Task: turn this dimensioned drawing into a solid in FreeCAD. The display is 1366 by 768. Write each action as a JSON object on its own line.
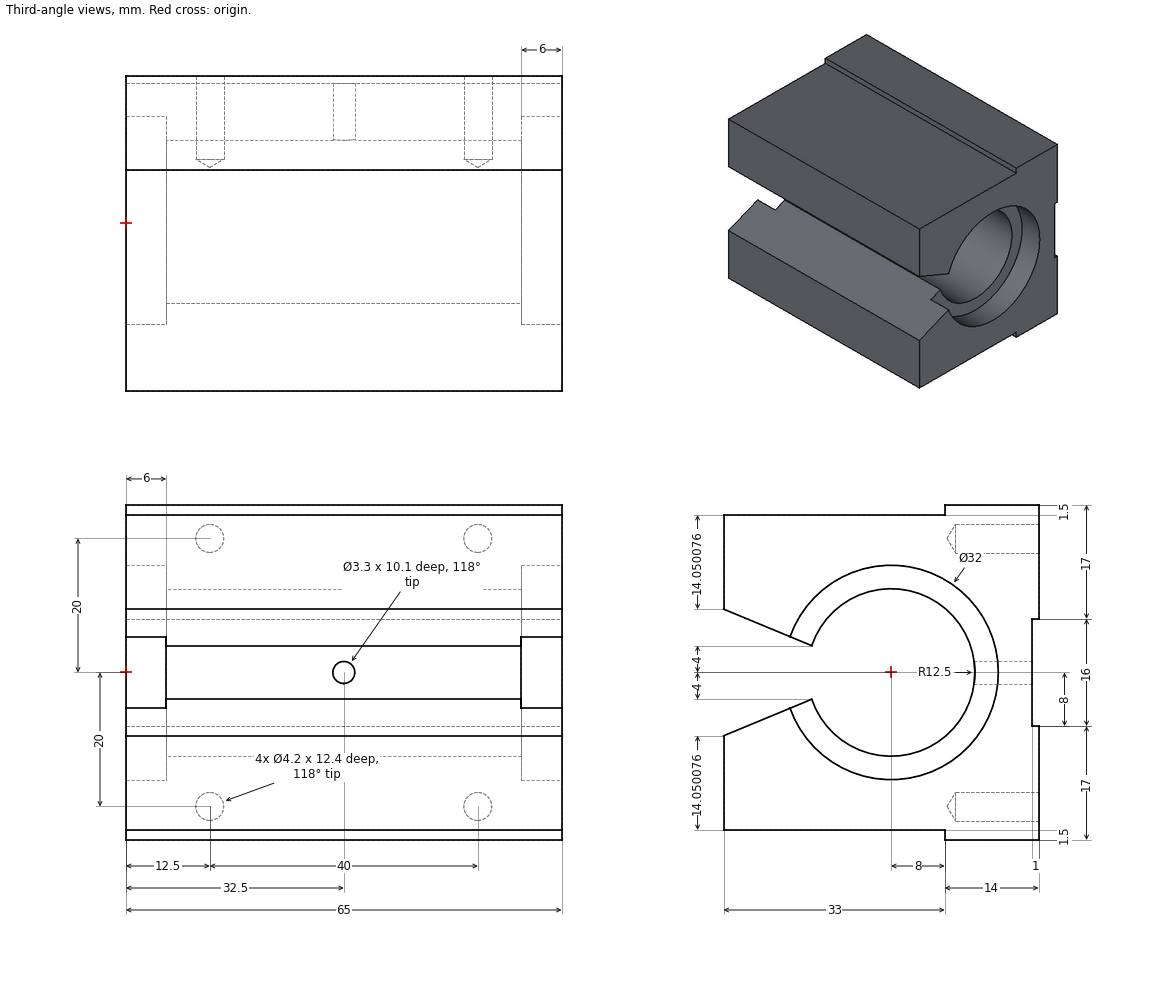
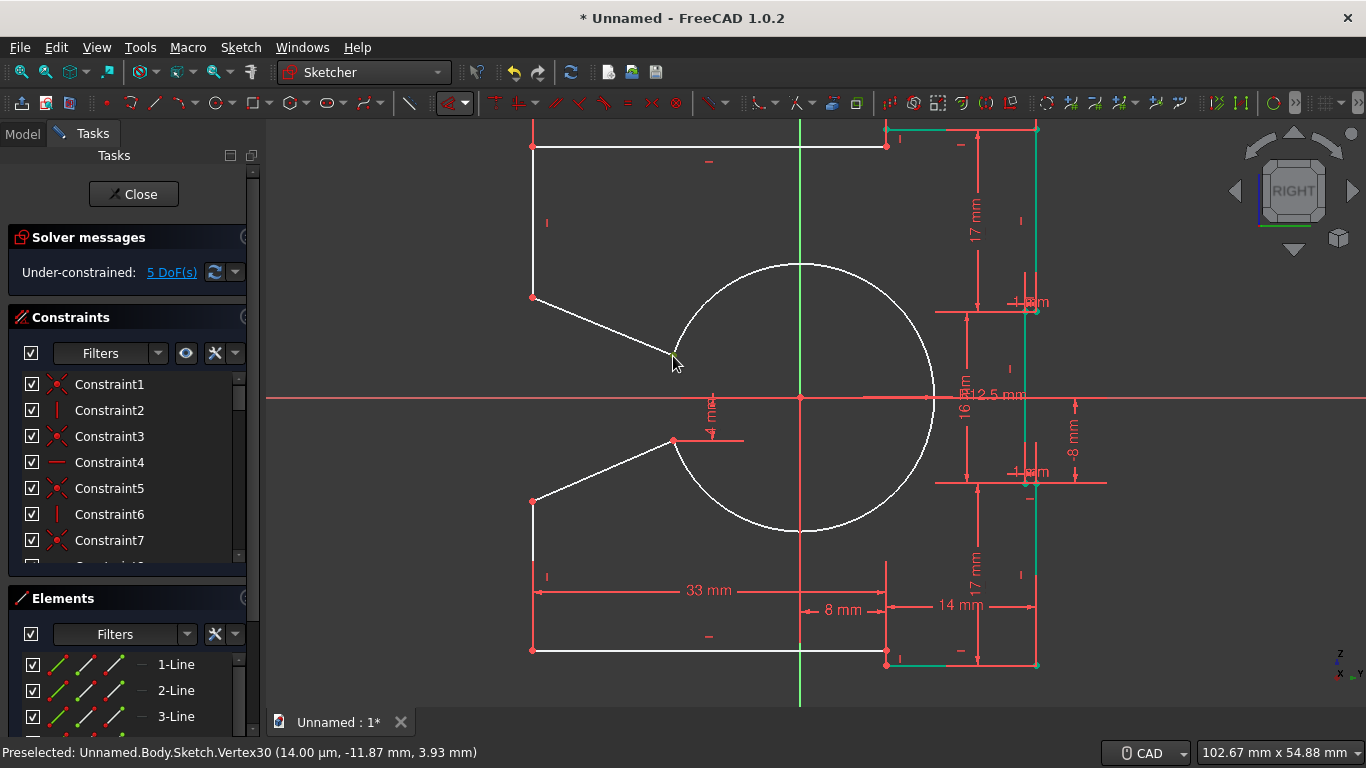
{"action": "key", "text": "i"}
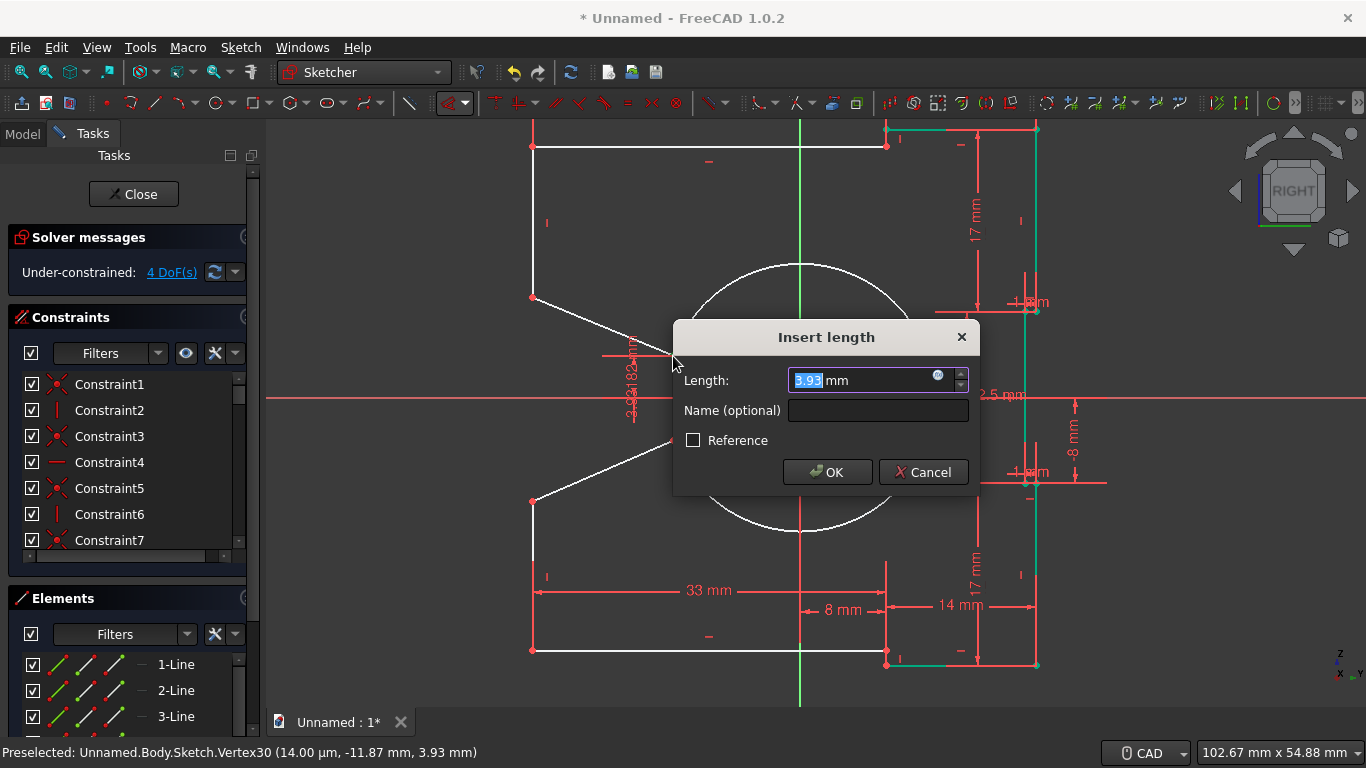
{"action": "type", "text": "4"}
{"action": "key", "text": "Return"}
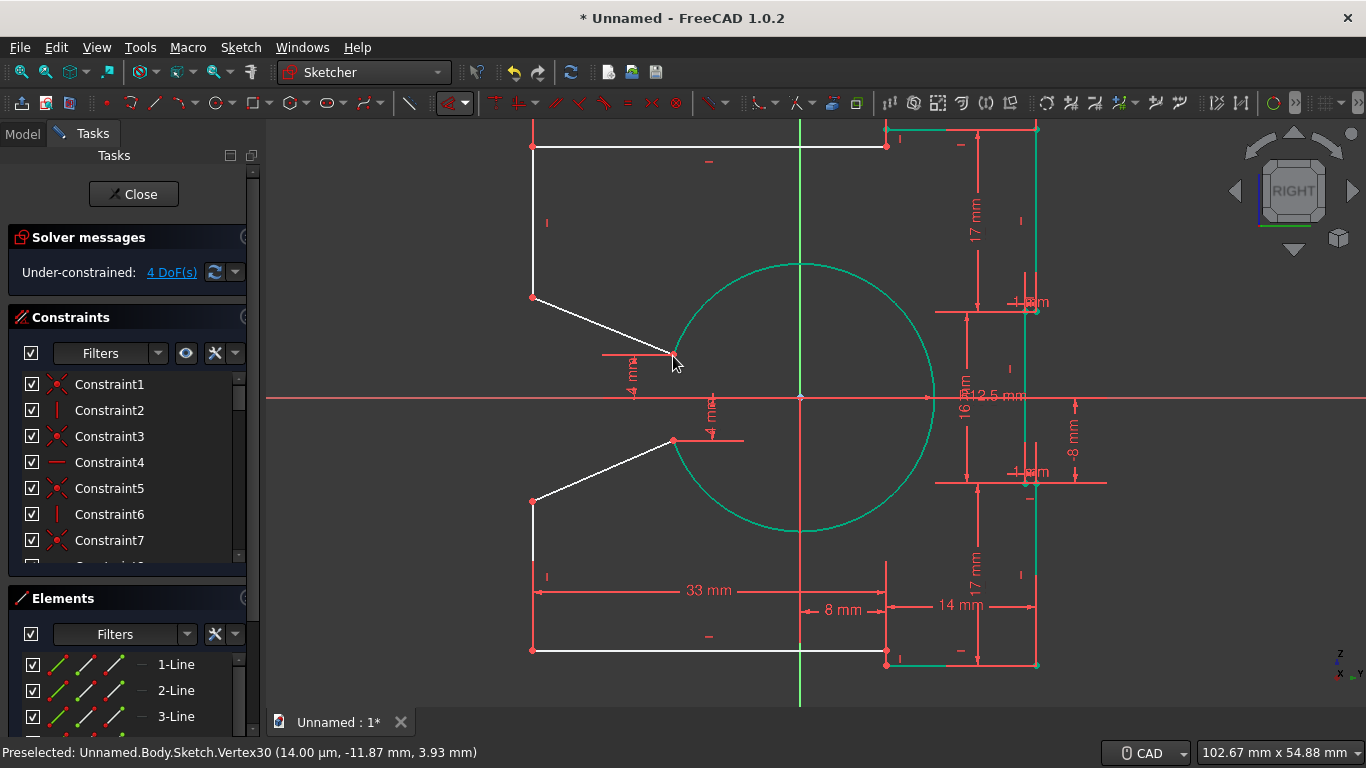
{"action": "scroll", "coordinate": [886, 658], "scroll_direction": "up", "scroll_amount": 5}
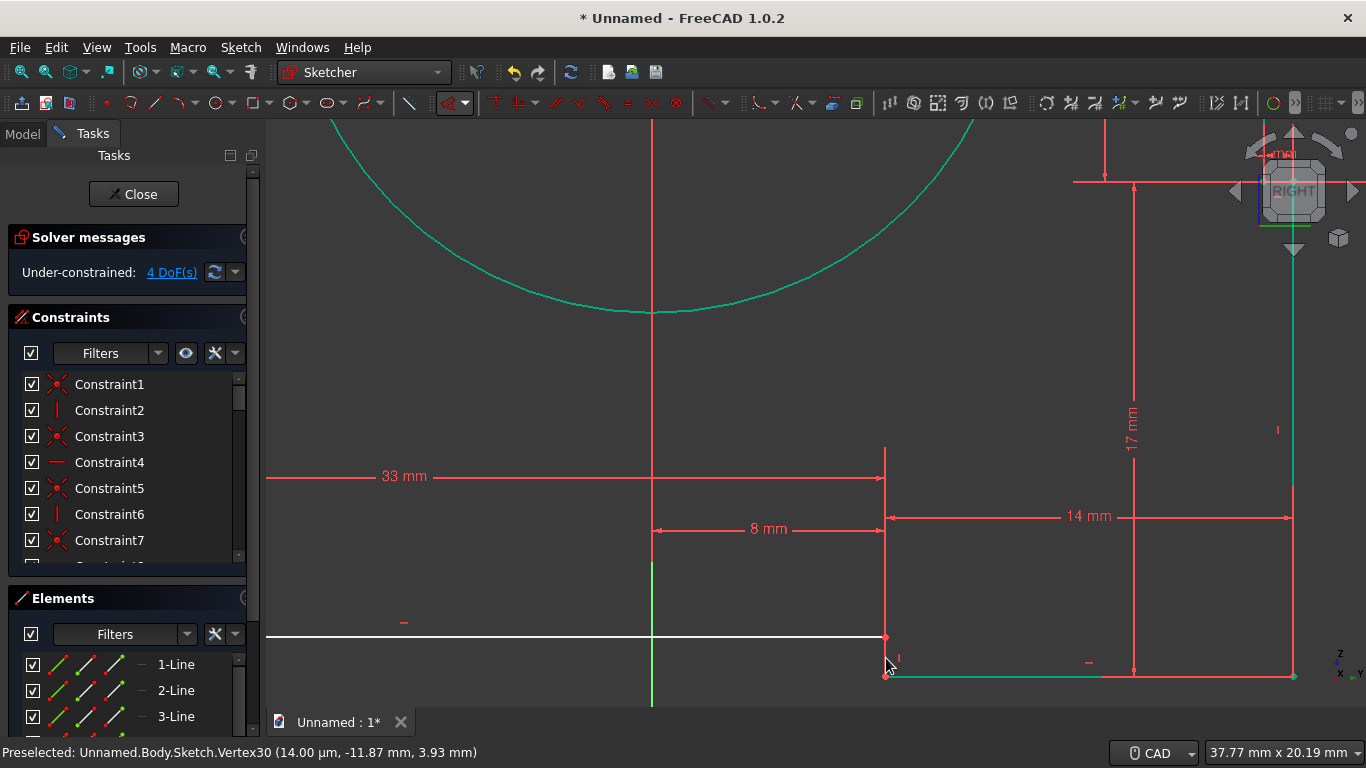
{"action": "left_click", "coordinate": [885, 657]}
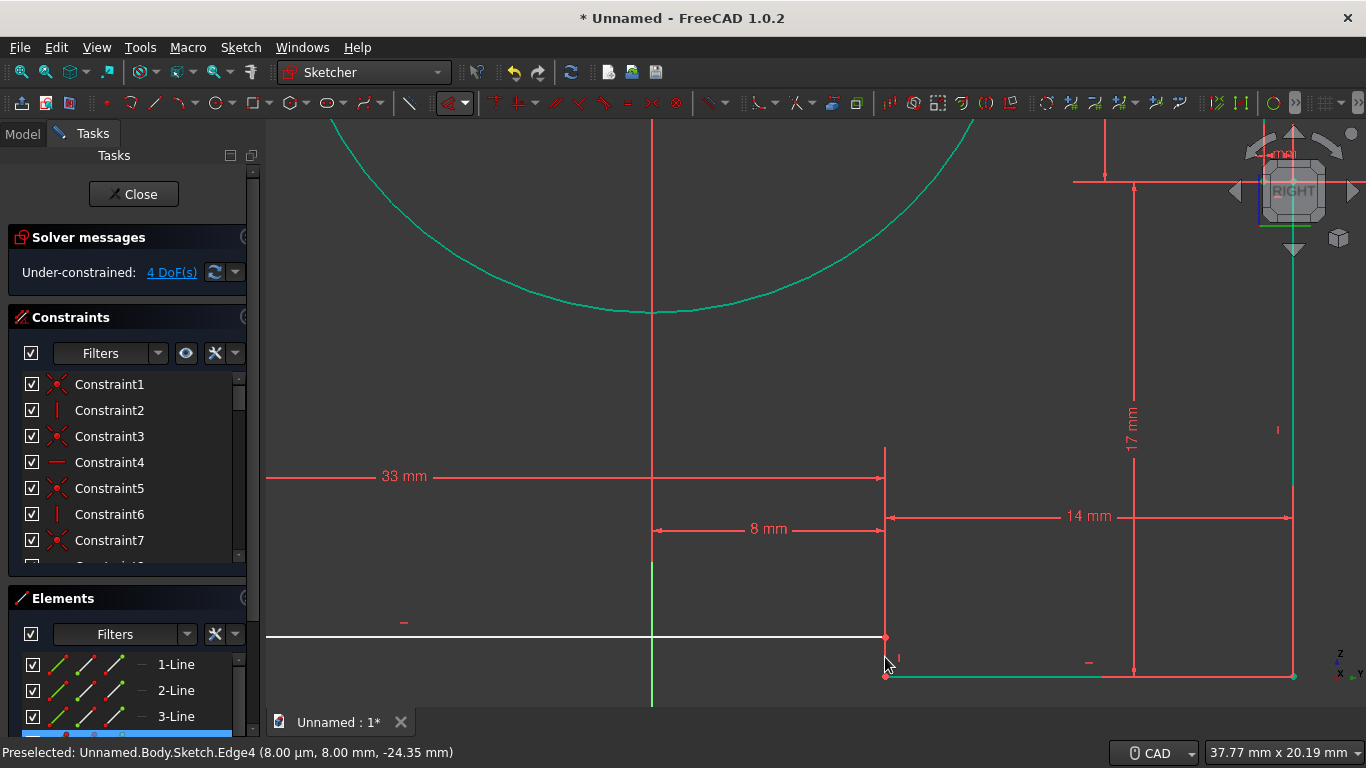
{"action": "left_click", "coordinate": [468, 104]}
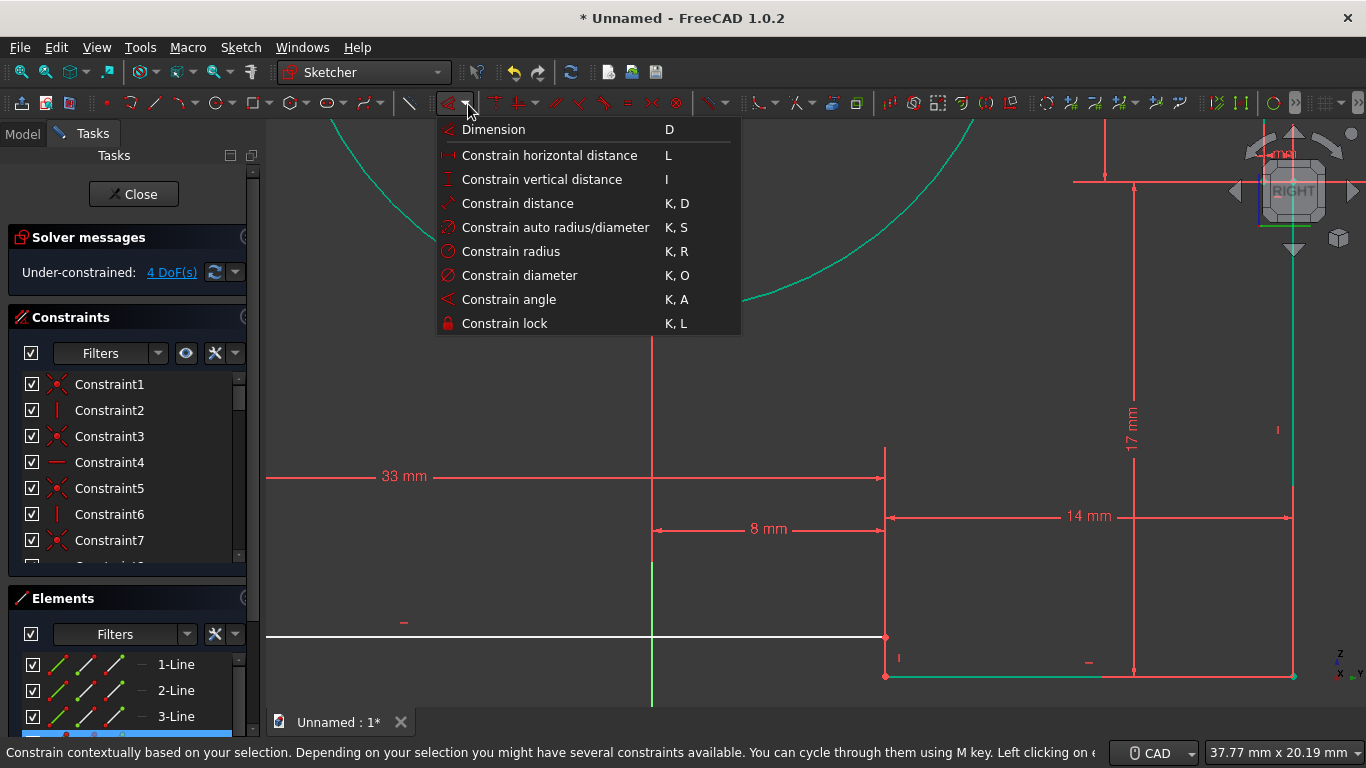
{"action": "left_click", "coordinate": [589, 179]}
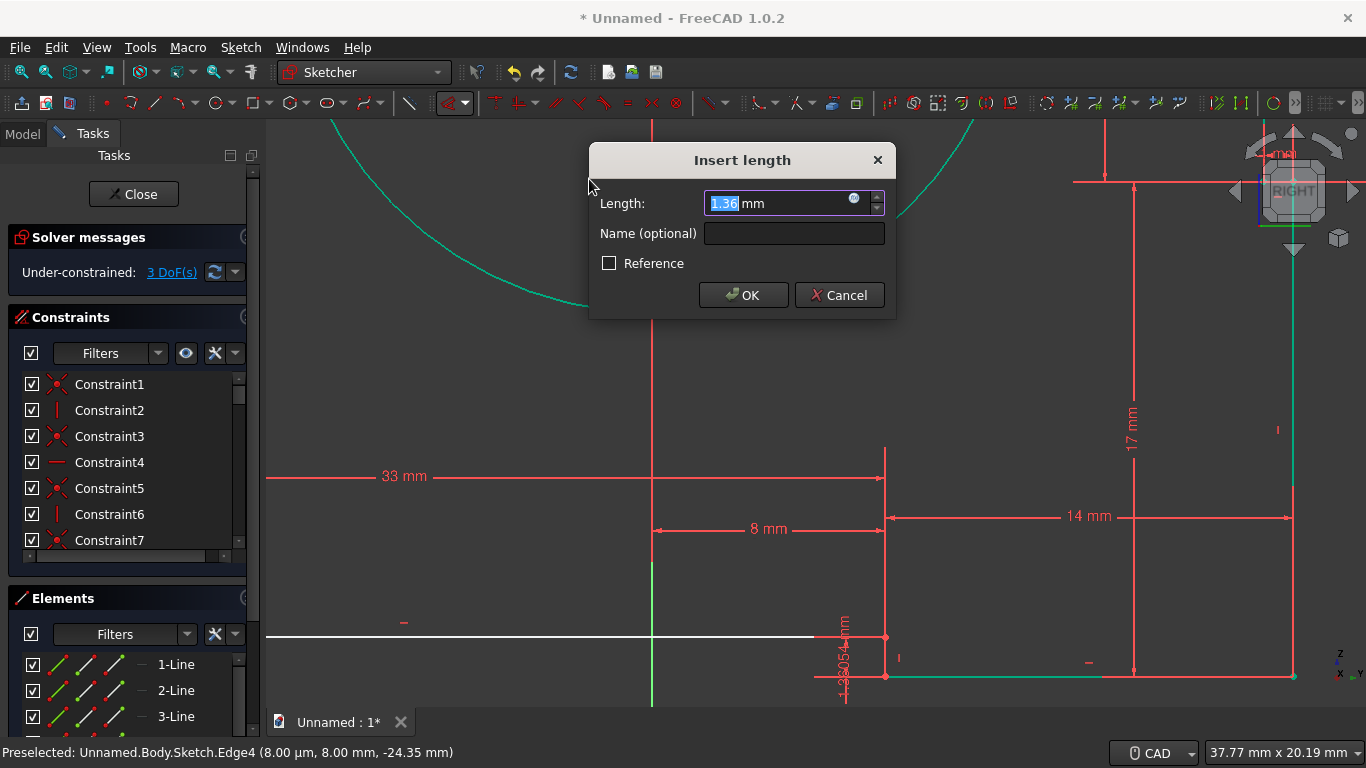
{"action": "type", "text": "1.5"}
{"action": "key", "text": "Return"}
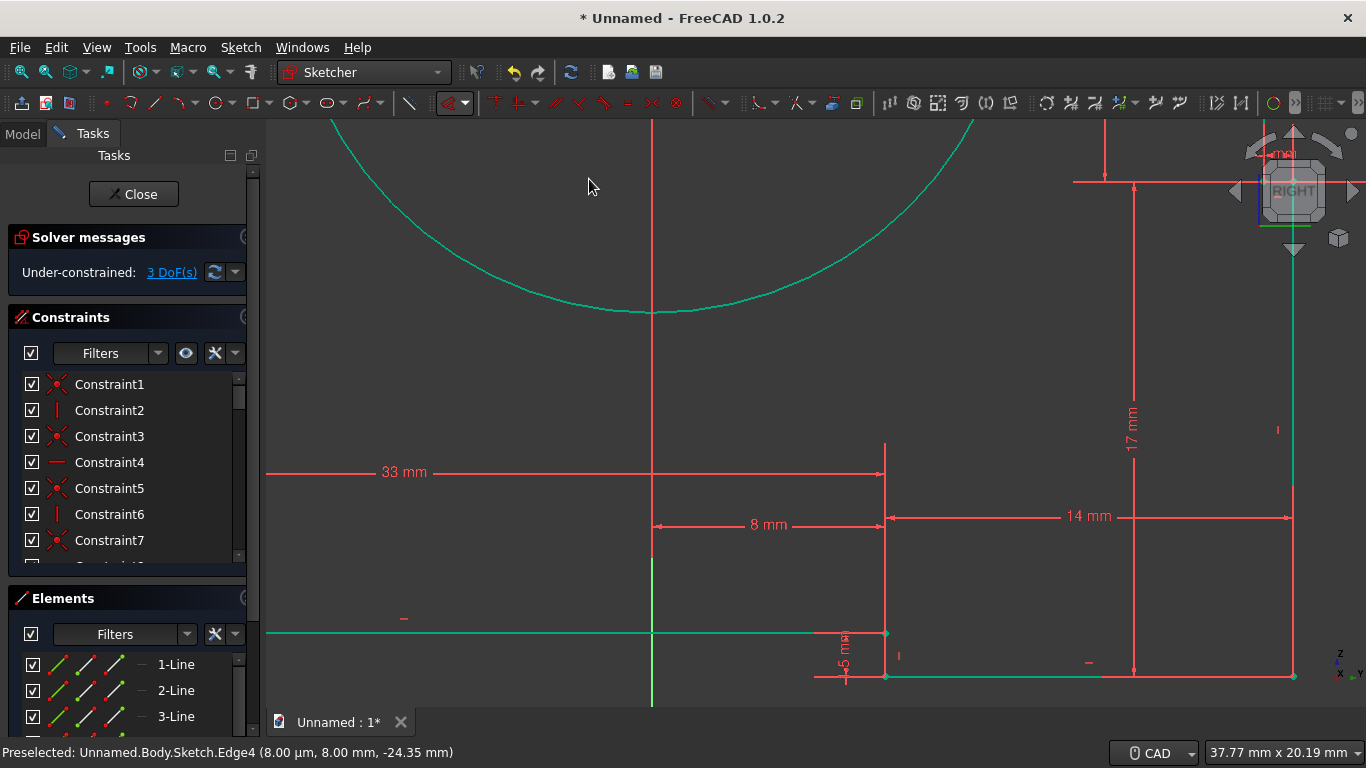
{"action": "scroll", "coordinate": [793, 565], "scroll_direction": "down", "scroll_amount": 7}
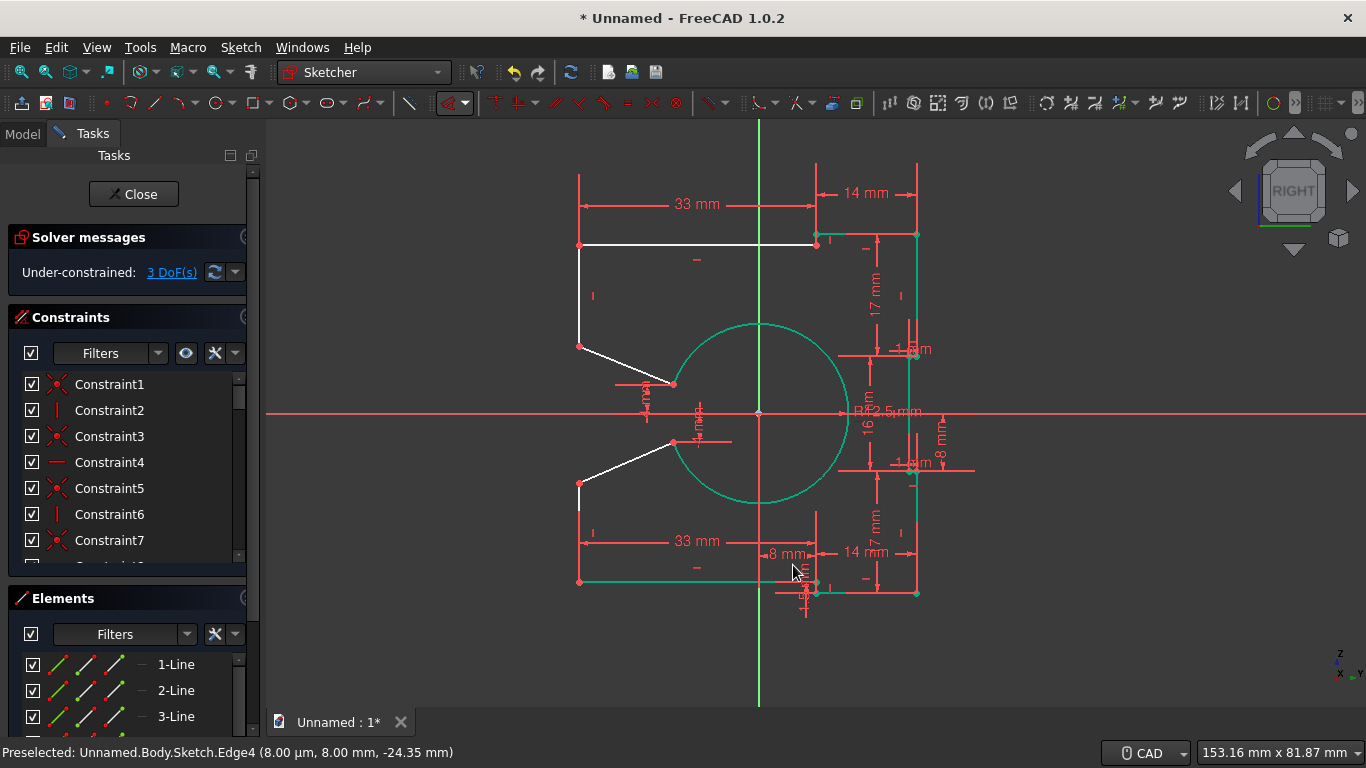
{"action": "scroll", "coordinate": [816, 237], "scroll_direction": "up", "scroll_amount": 8}